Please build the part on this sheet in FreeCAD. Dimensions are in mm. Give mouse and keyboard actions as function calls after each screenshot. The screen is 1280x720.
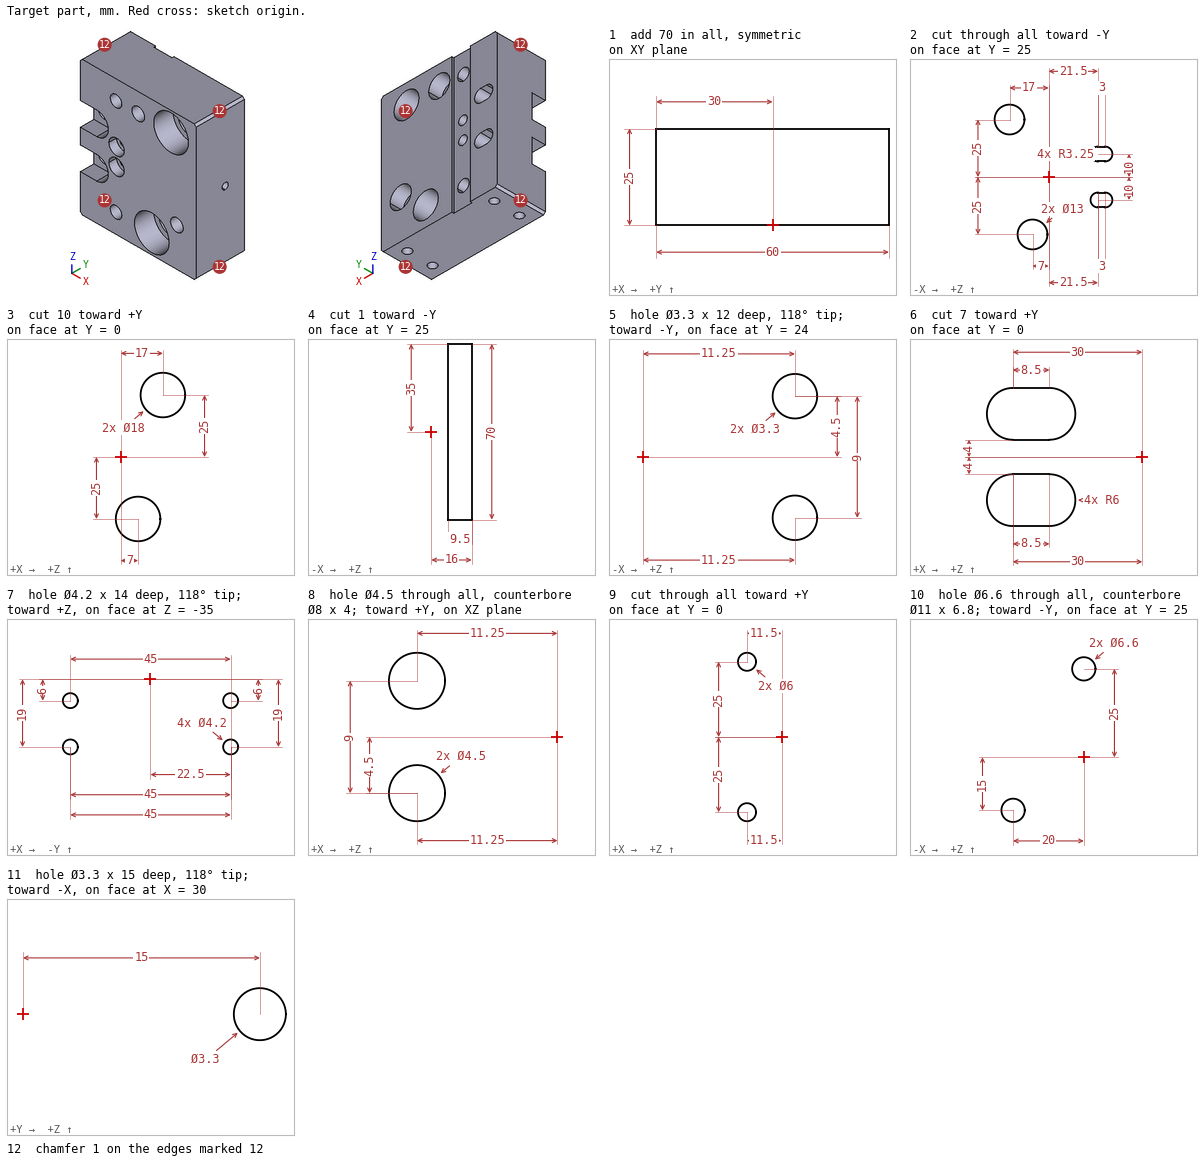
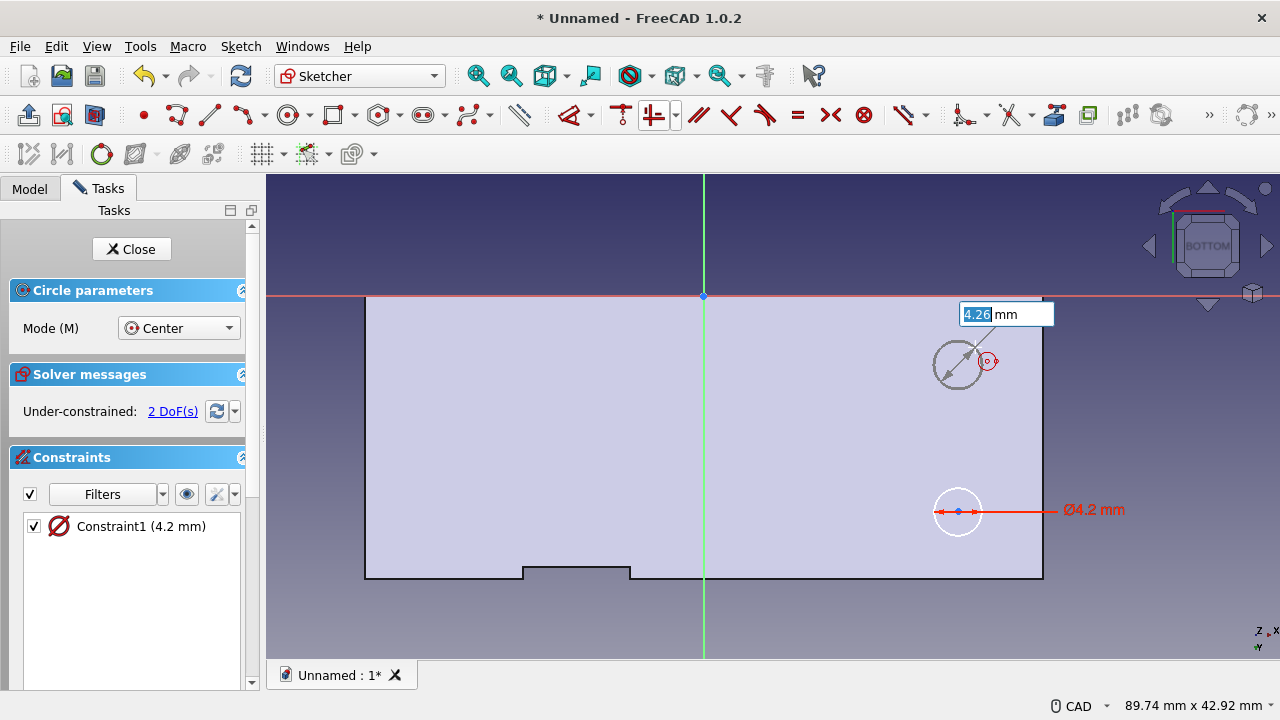
text(4.2)
key(Return)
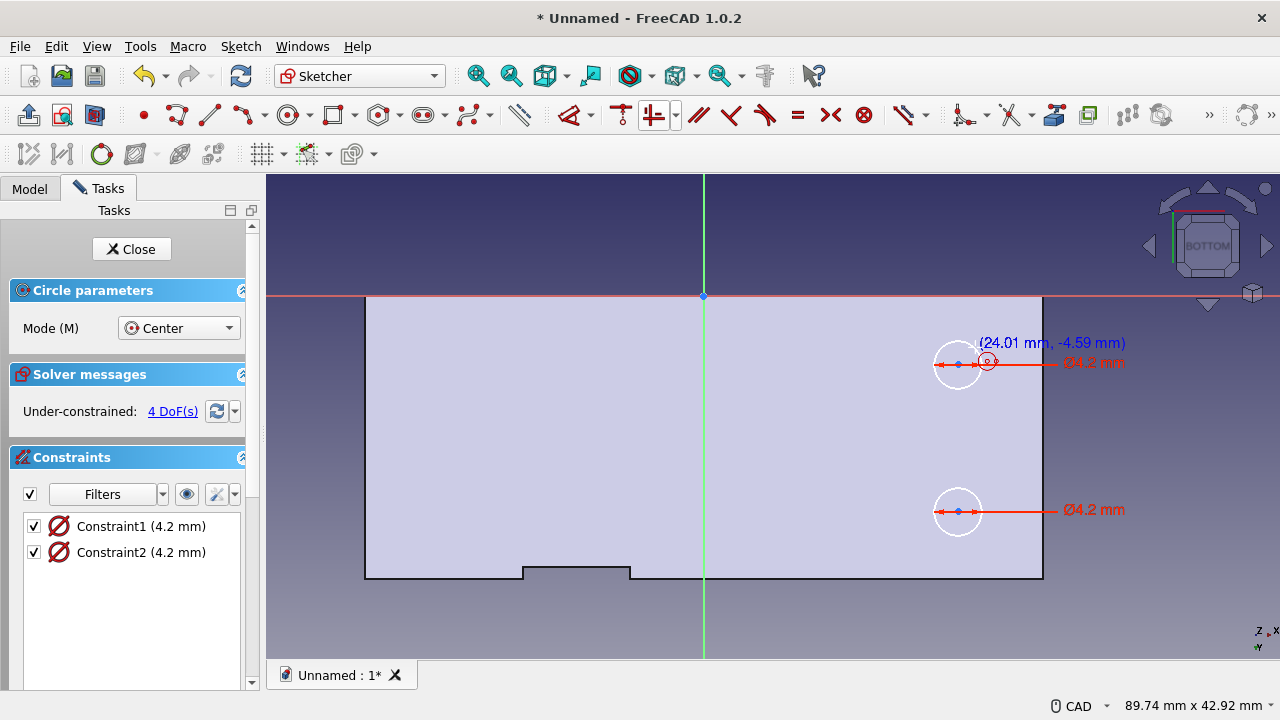
click(449, 511)
move(466, 494)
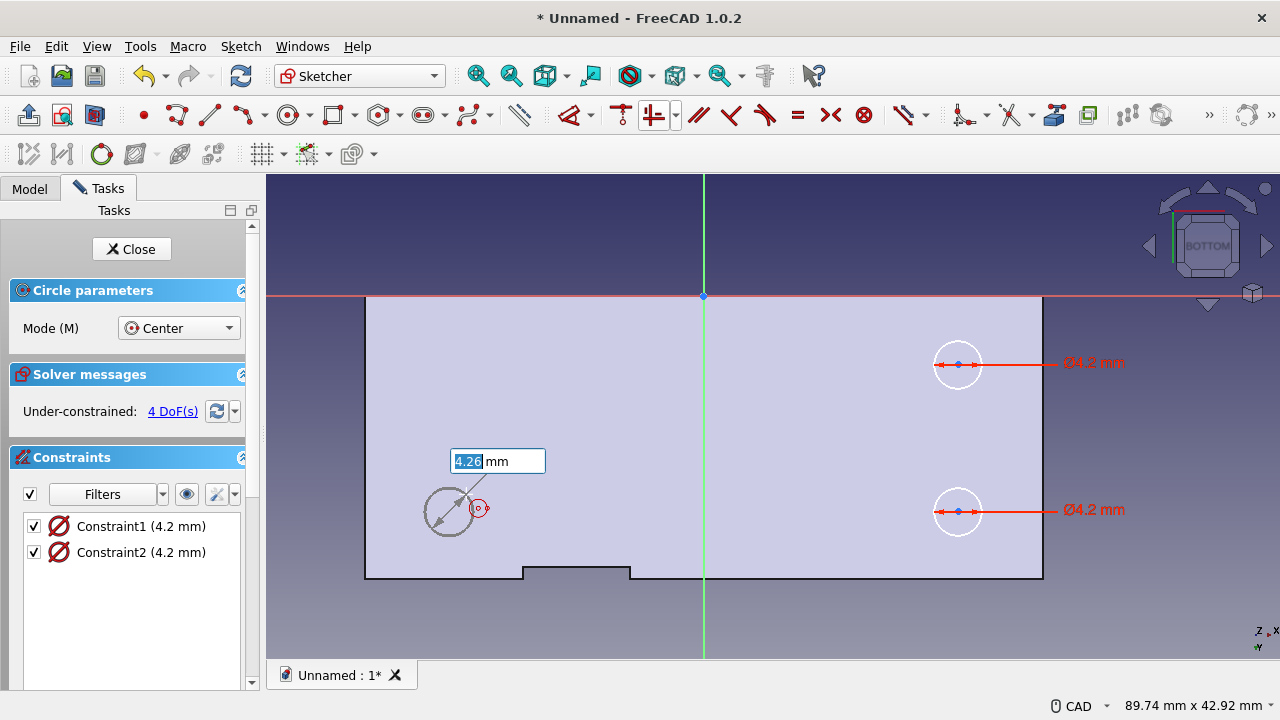
text(4.2)
key(Return)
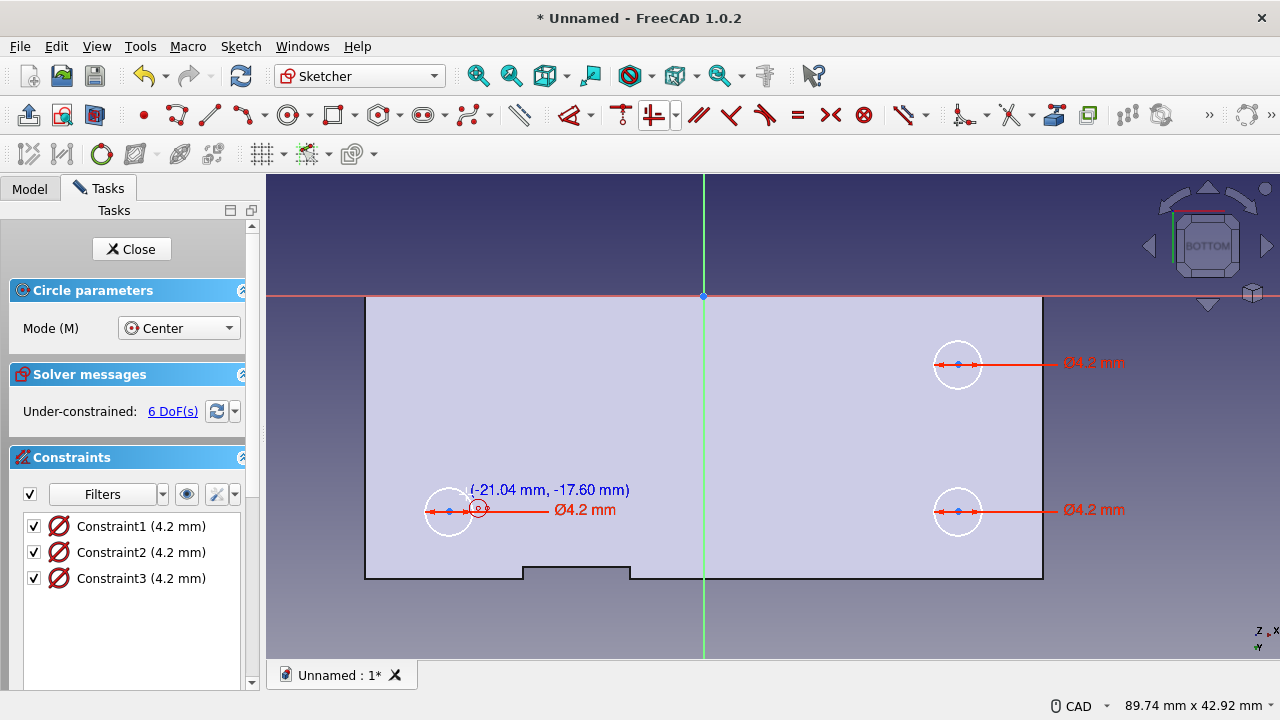
click(449, 364)
move(466, 347)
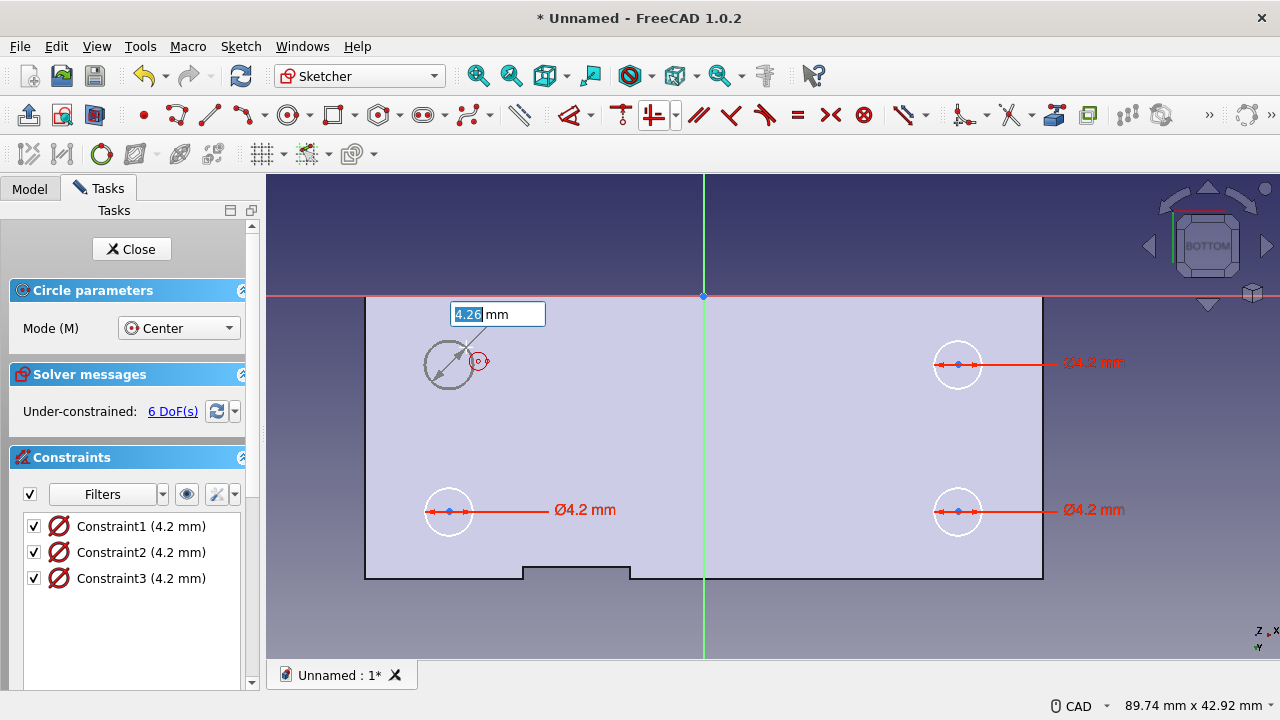
text(4.2)
key(Return)
key(Escape)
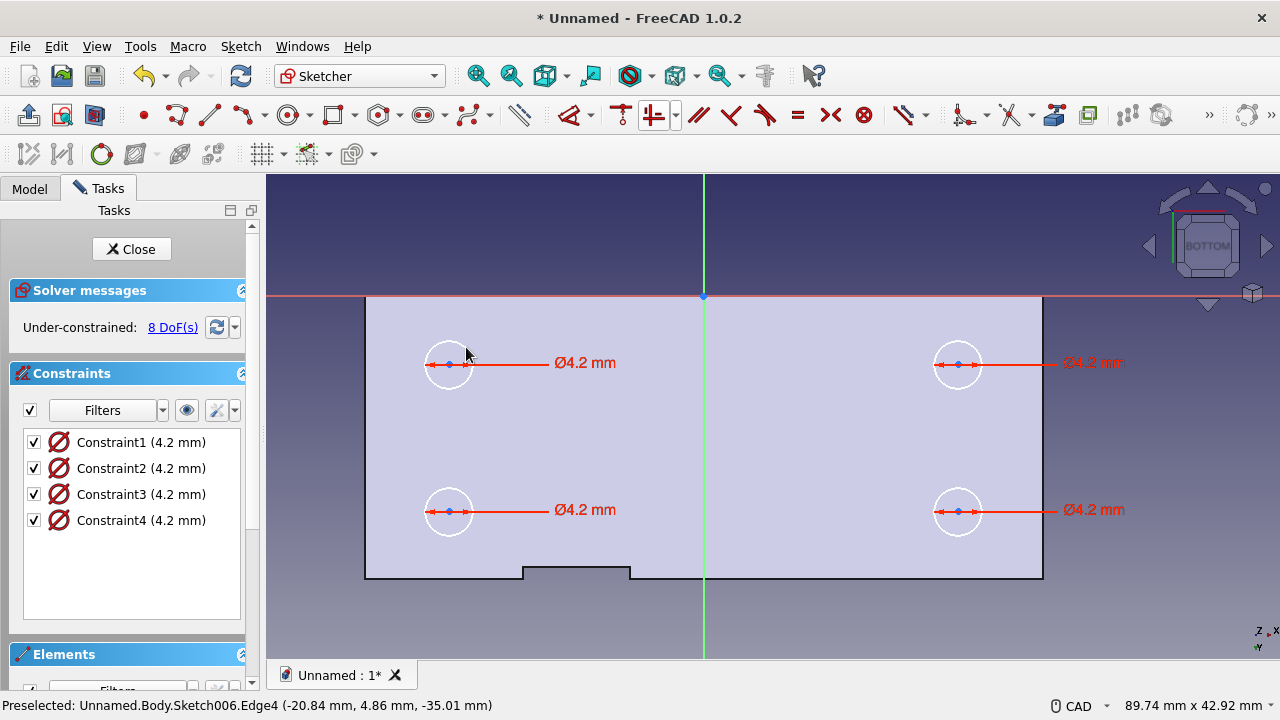
click(568, 116)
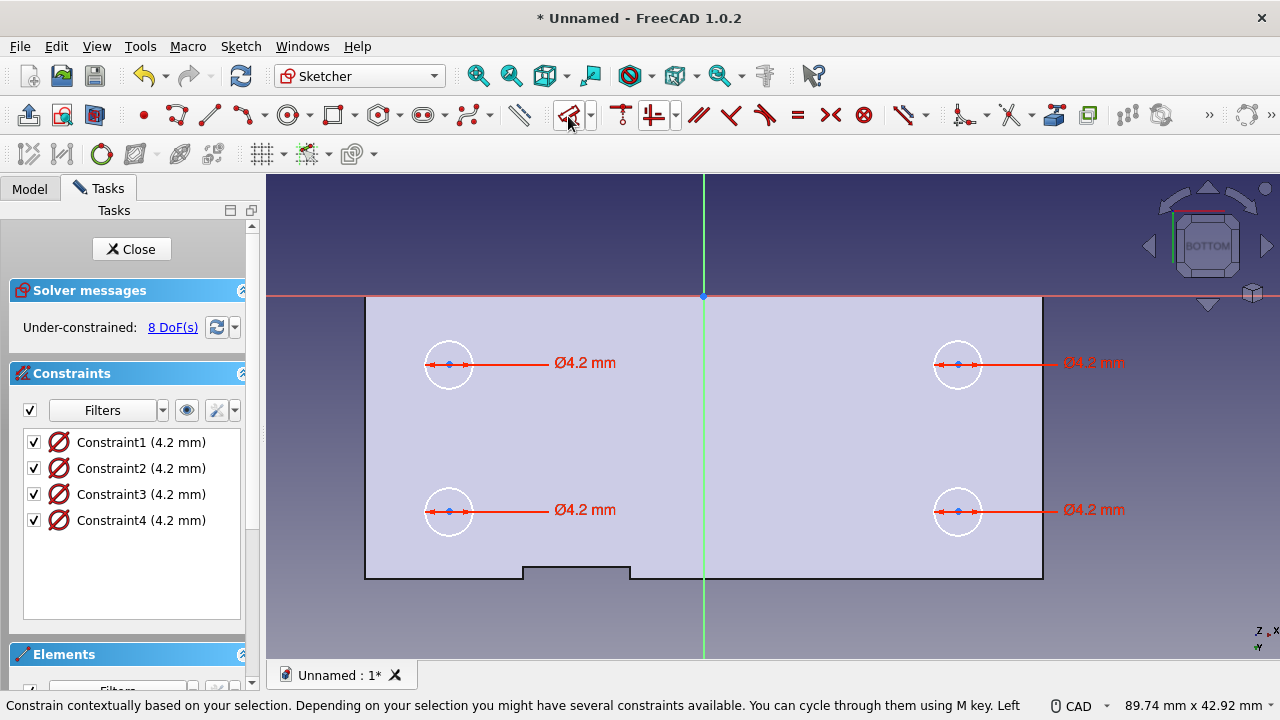
click(958, 365)
click(992, 331)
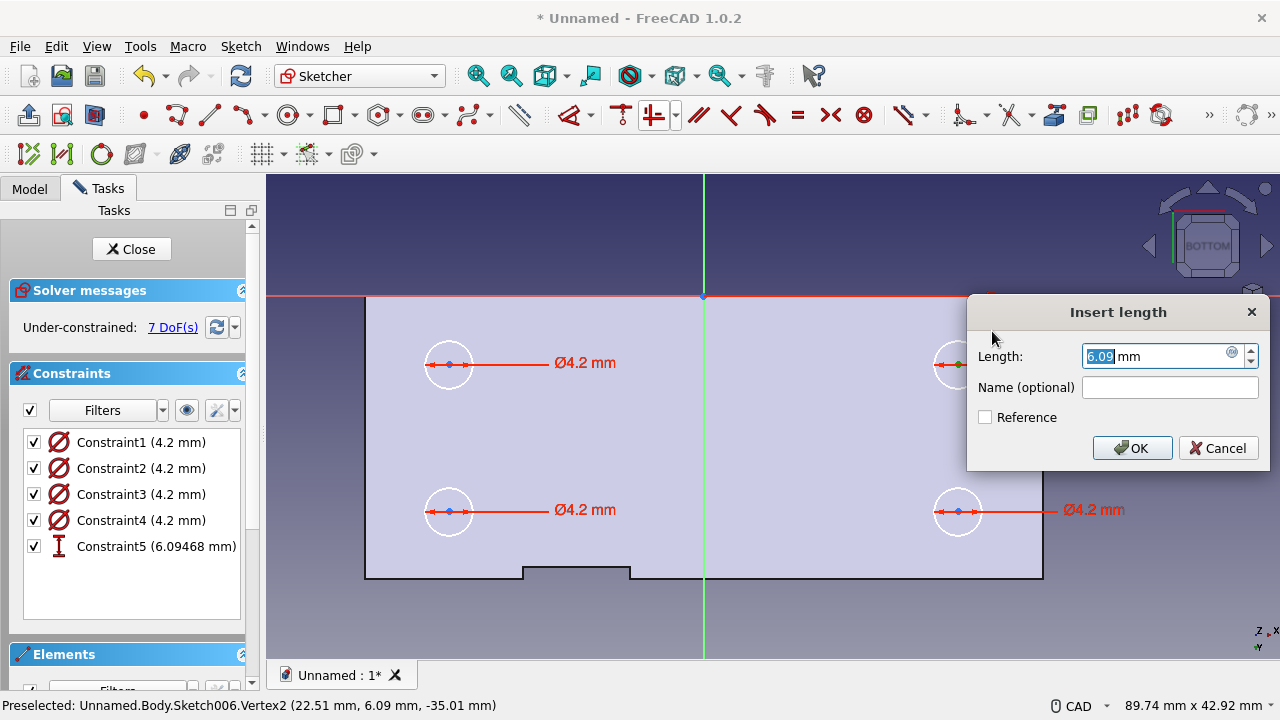
text(6)
key(Return)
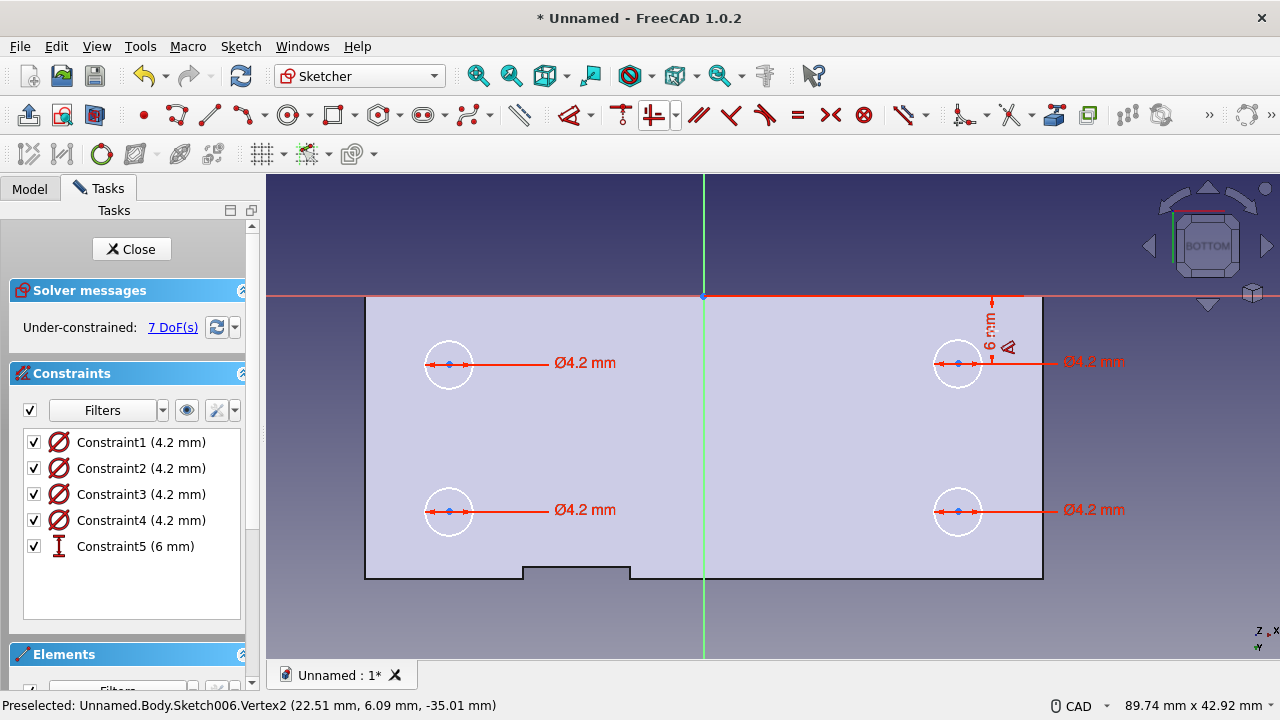
click(449, 365)
click(415, 331)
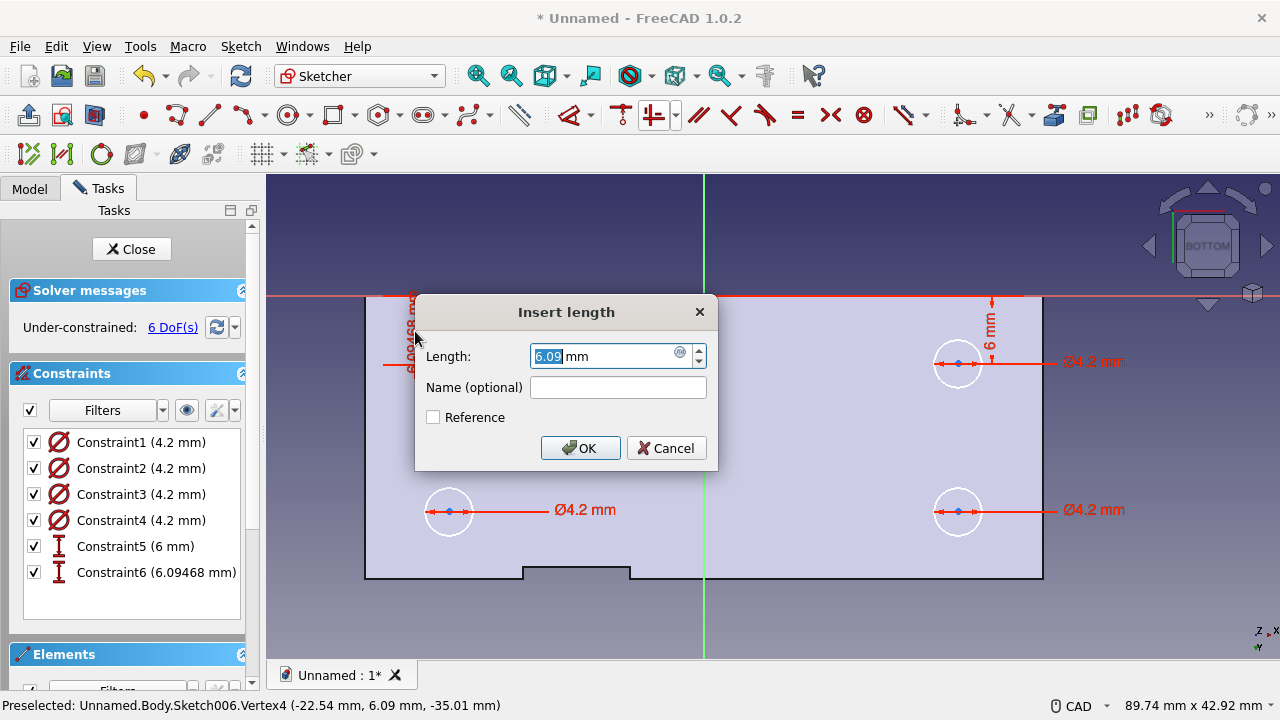
text(6)
key(Return)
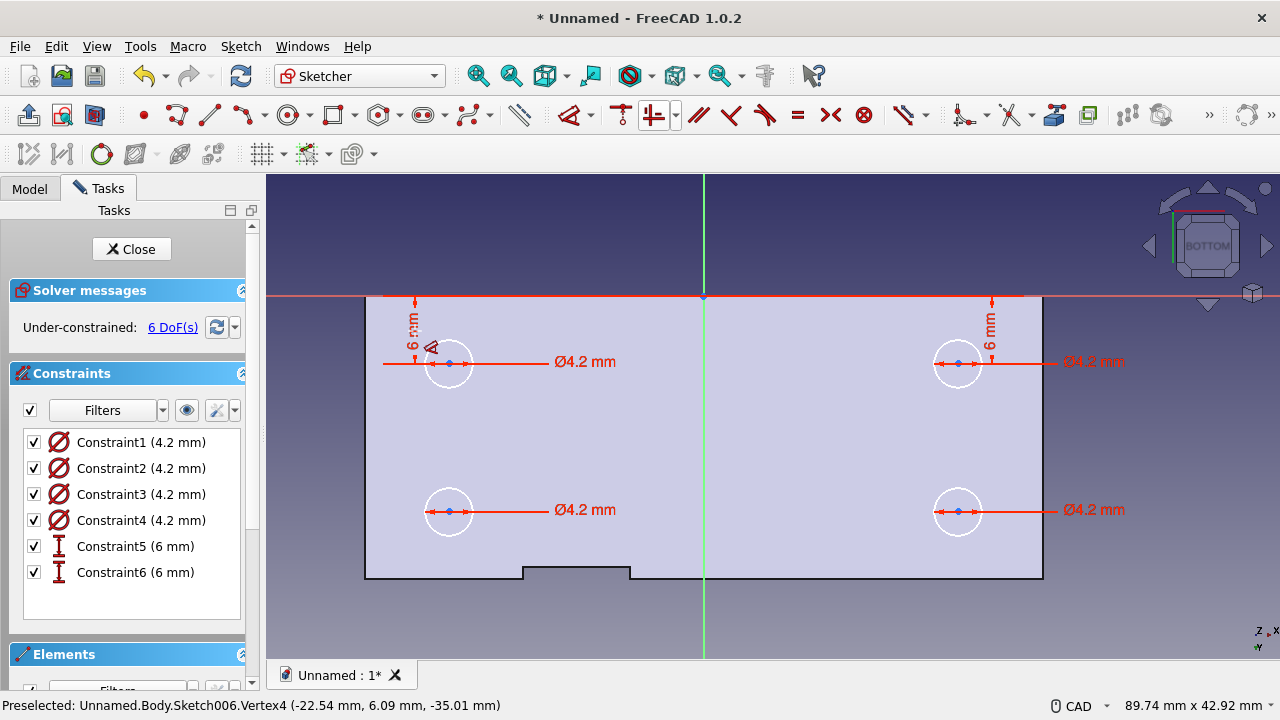
click(958, 512)
click(992, 404)